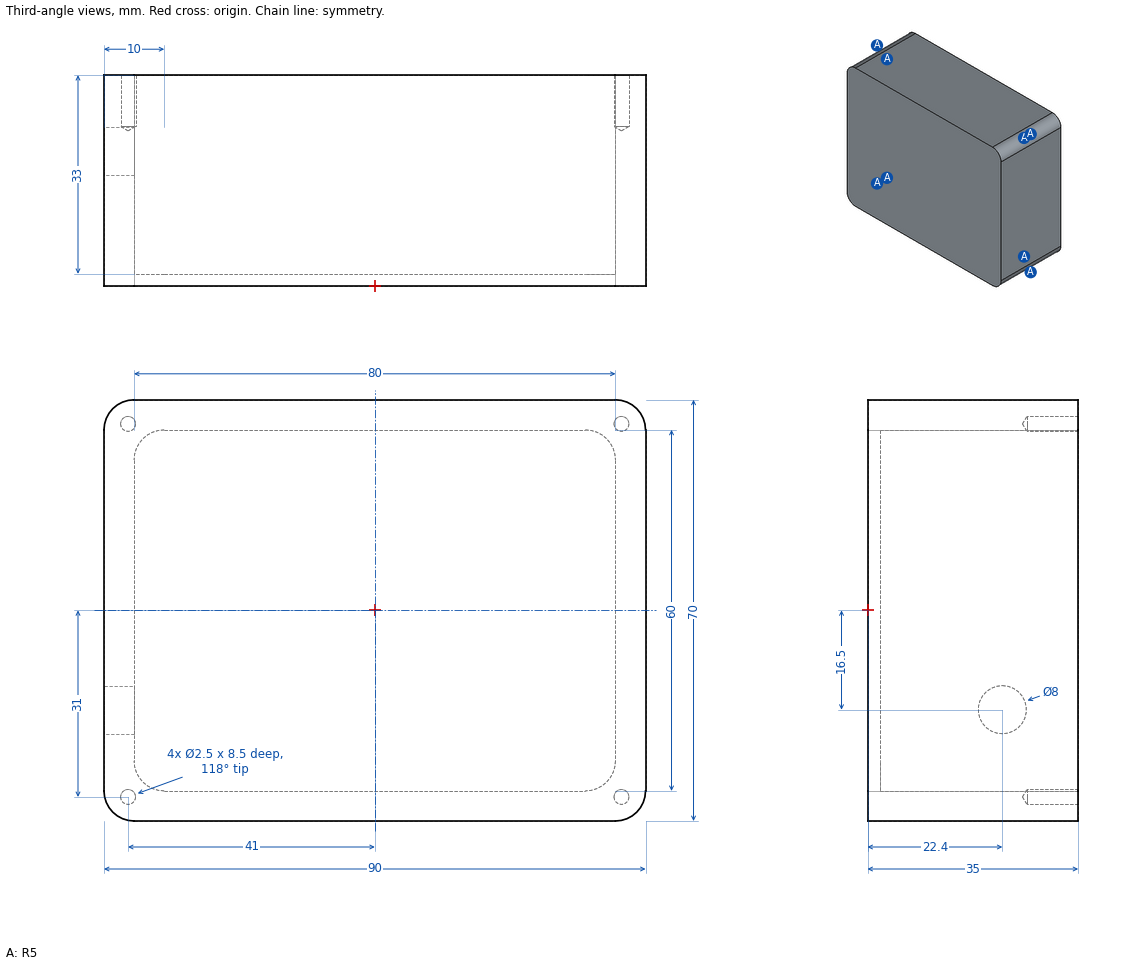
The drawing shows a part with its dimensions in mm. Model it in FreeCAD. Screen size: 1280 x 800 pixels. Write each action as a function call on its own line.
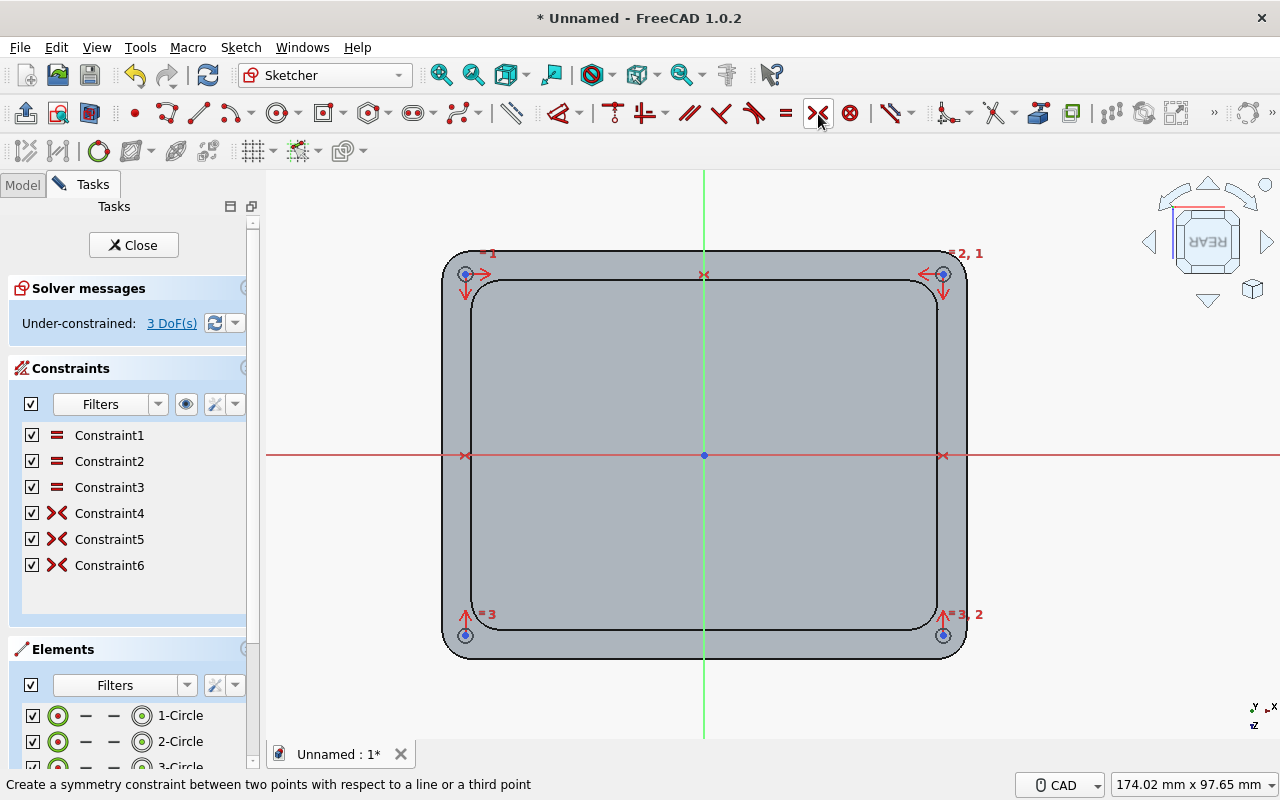
scroll(471, 279, up, 6)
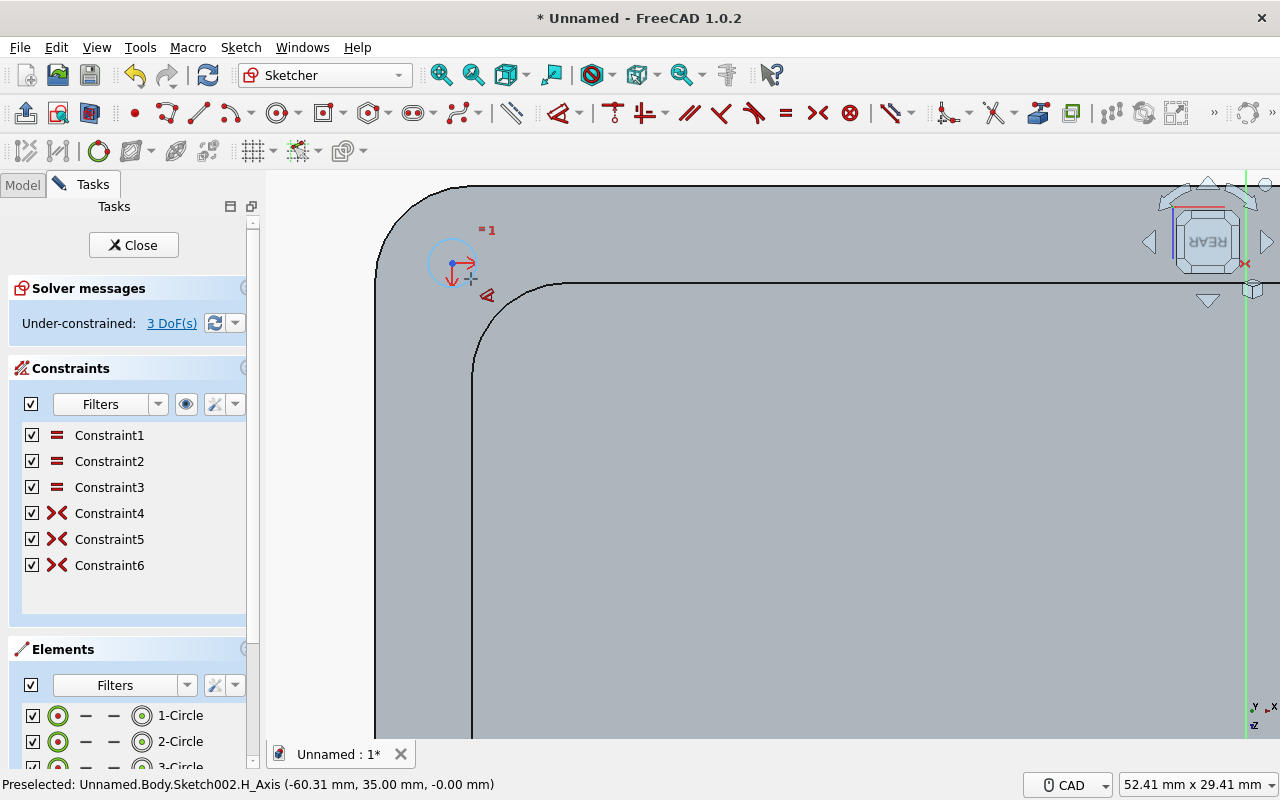
click(469, 280)
click(491, 303)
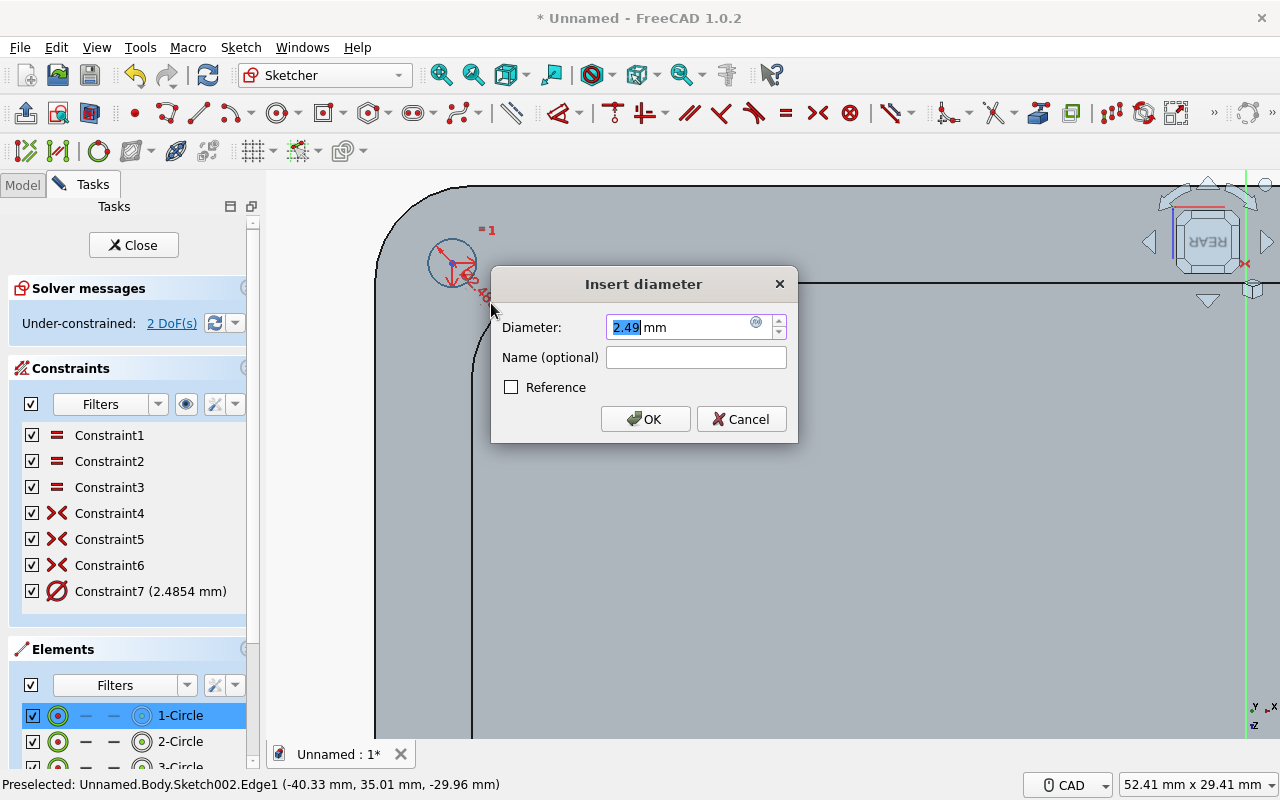
text(2.5)
key(Return)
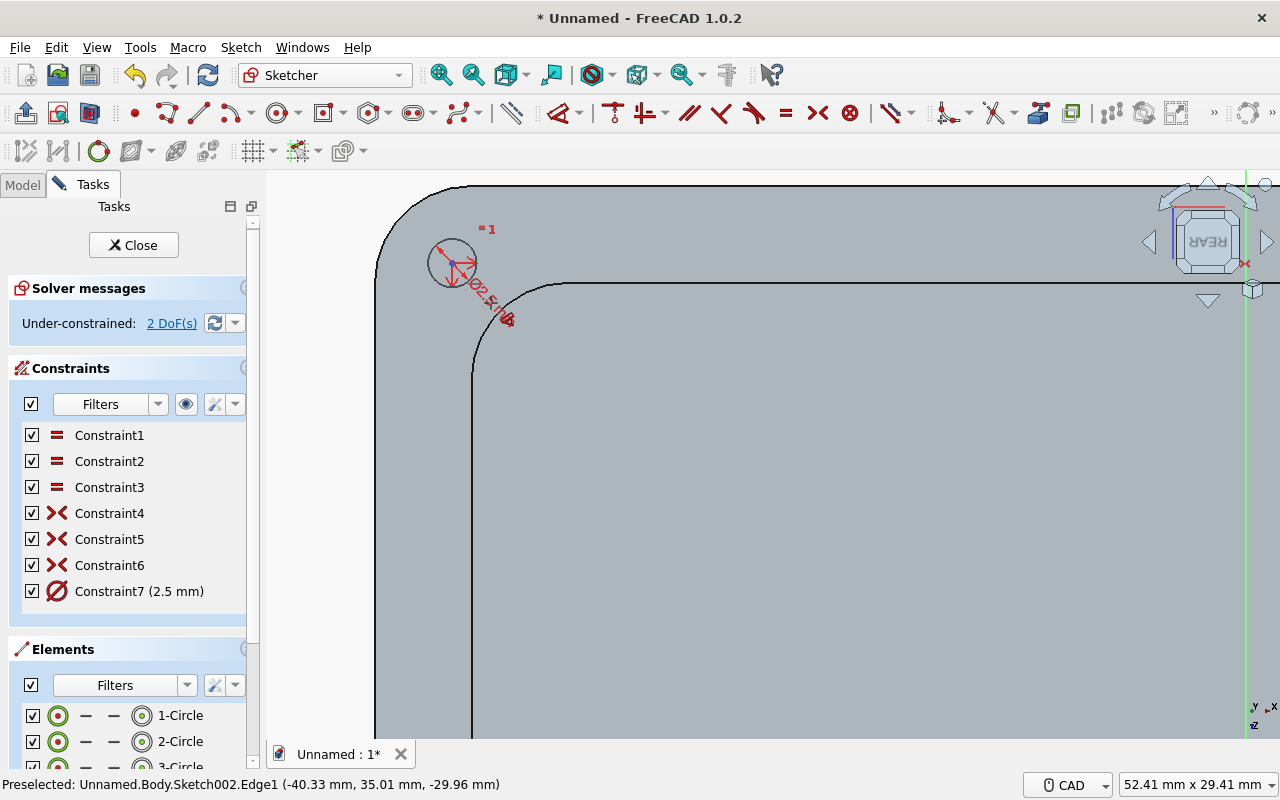
click(452, 263)
click(784, 229)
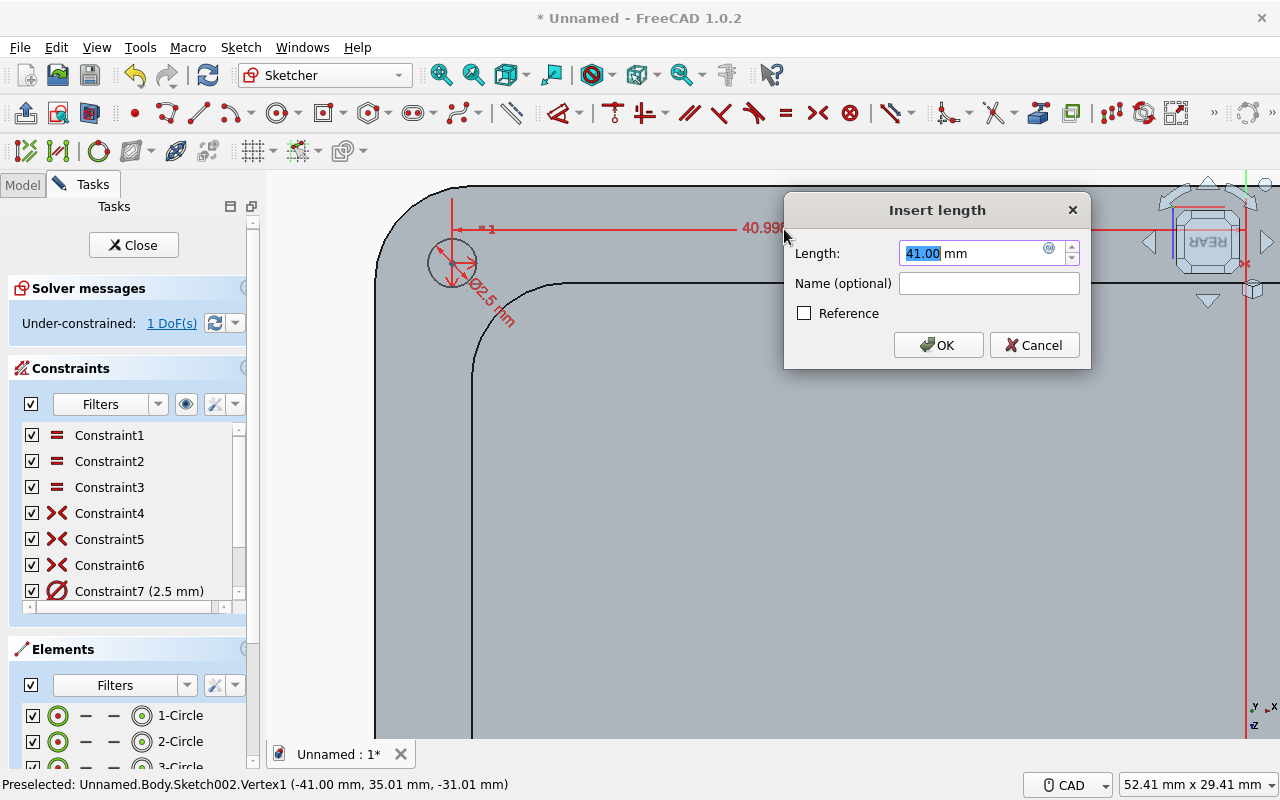
text(41)
key(Return)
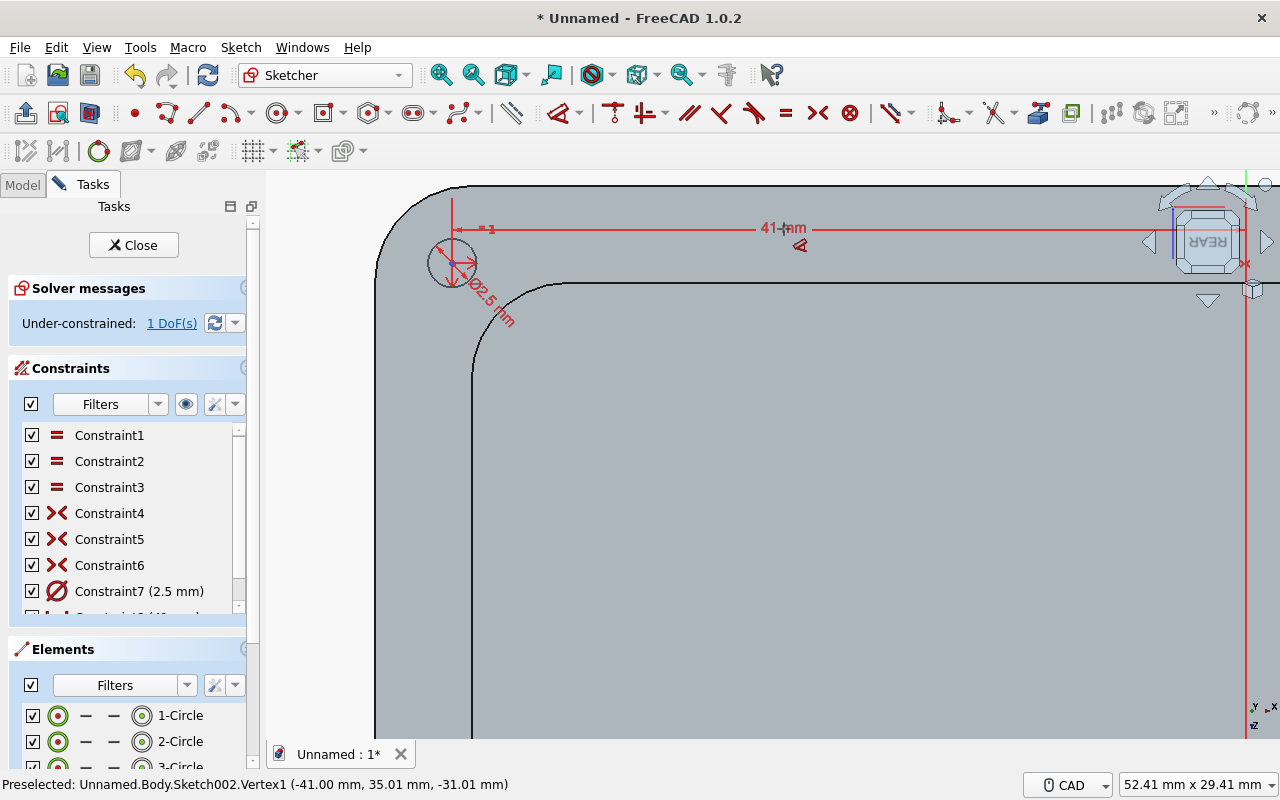
click(452, 263)
click(418, 487)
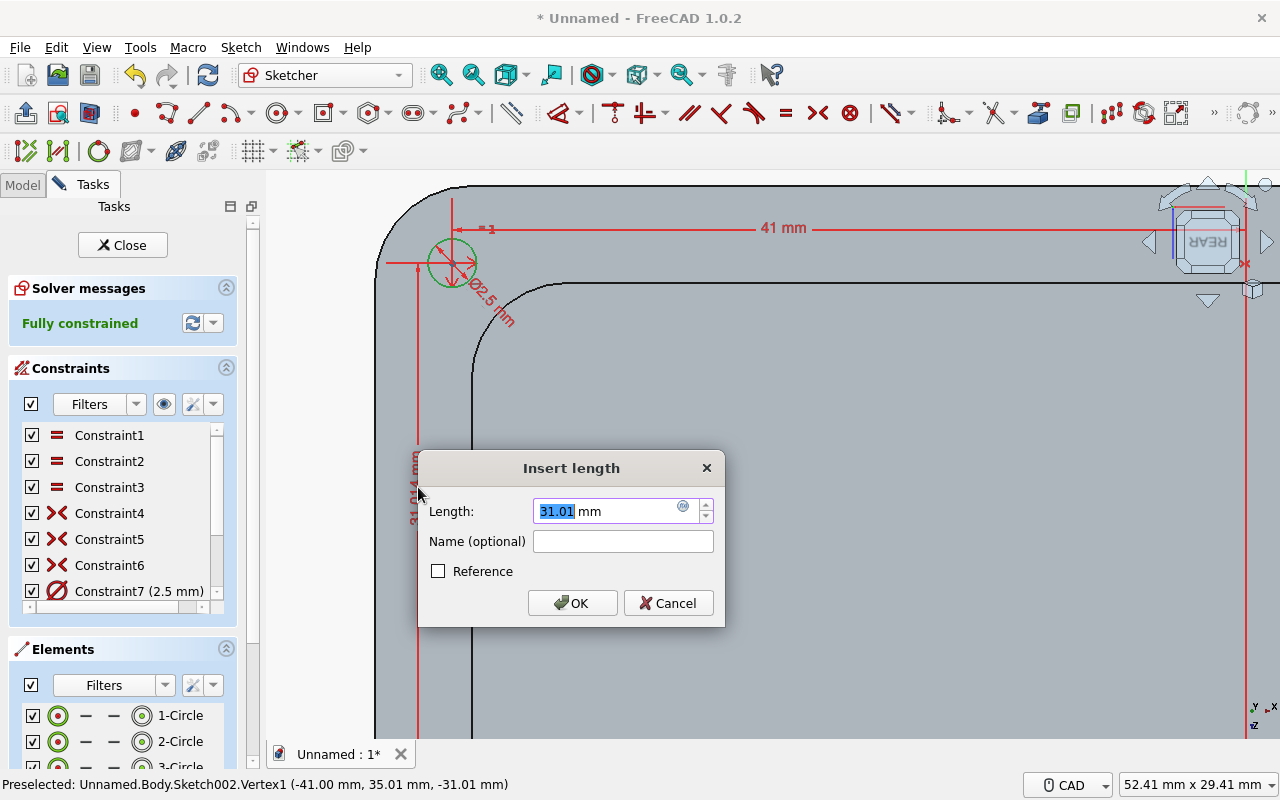
text(31)
key(Return)
key(Escape)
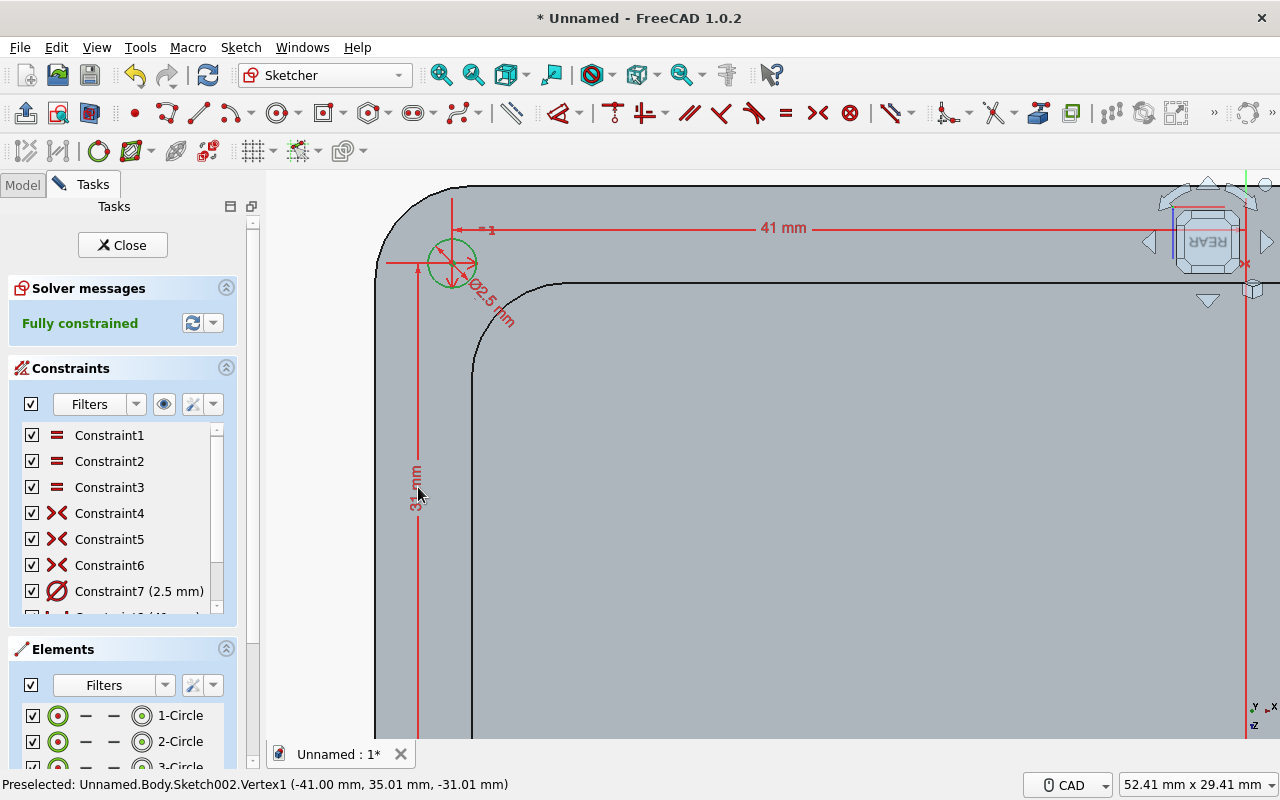
click(123, 245)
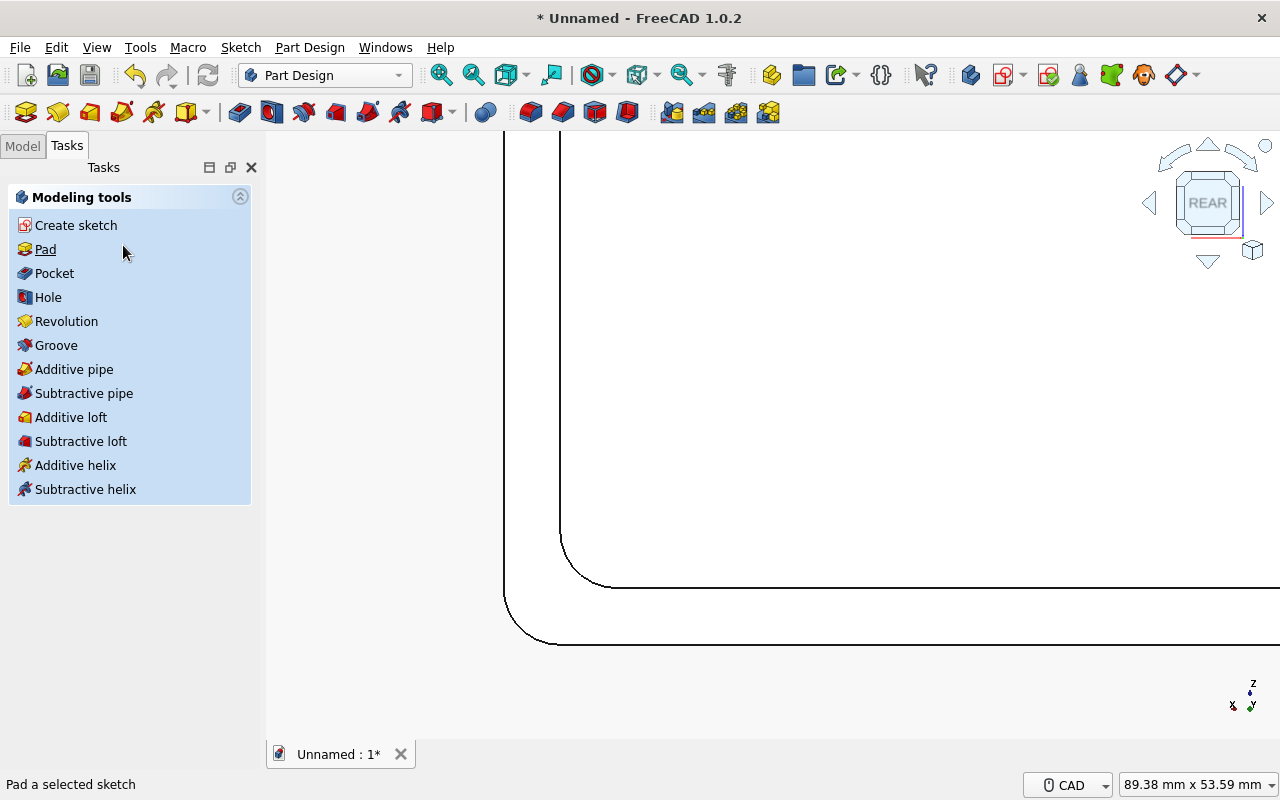
click(272, 112)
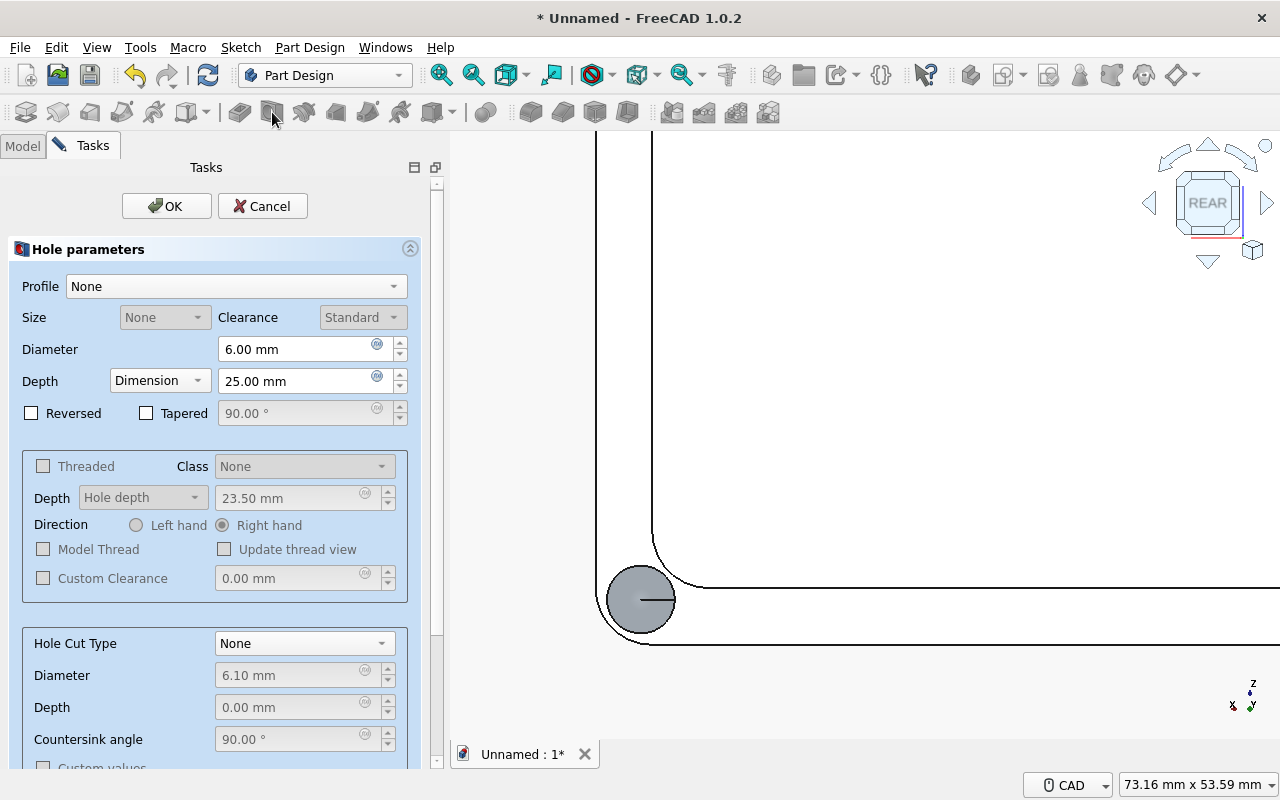
triple_click(305, 349)